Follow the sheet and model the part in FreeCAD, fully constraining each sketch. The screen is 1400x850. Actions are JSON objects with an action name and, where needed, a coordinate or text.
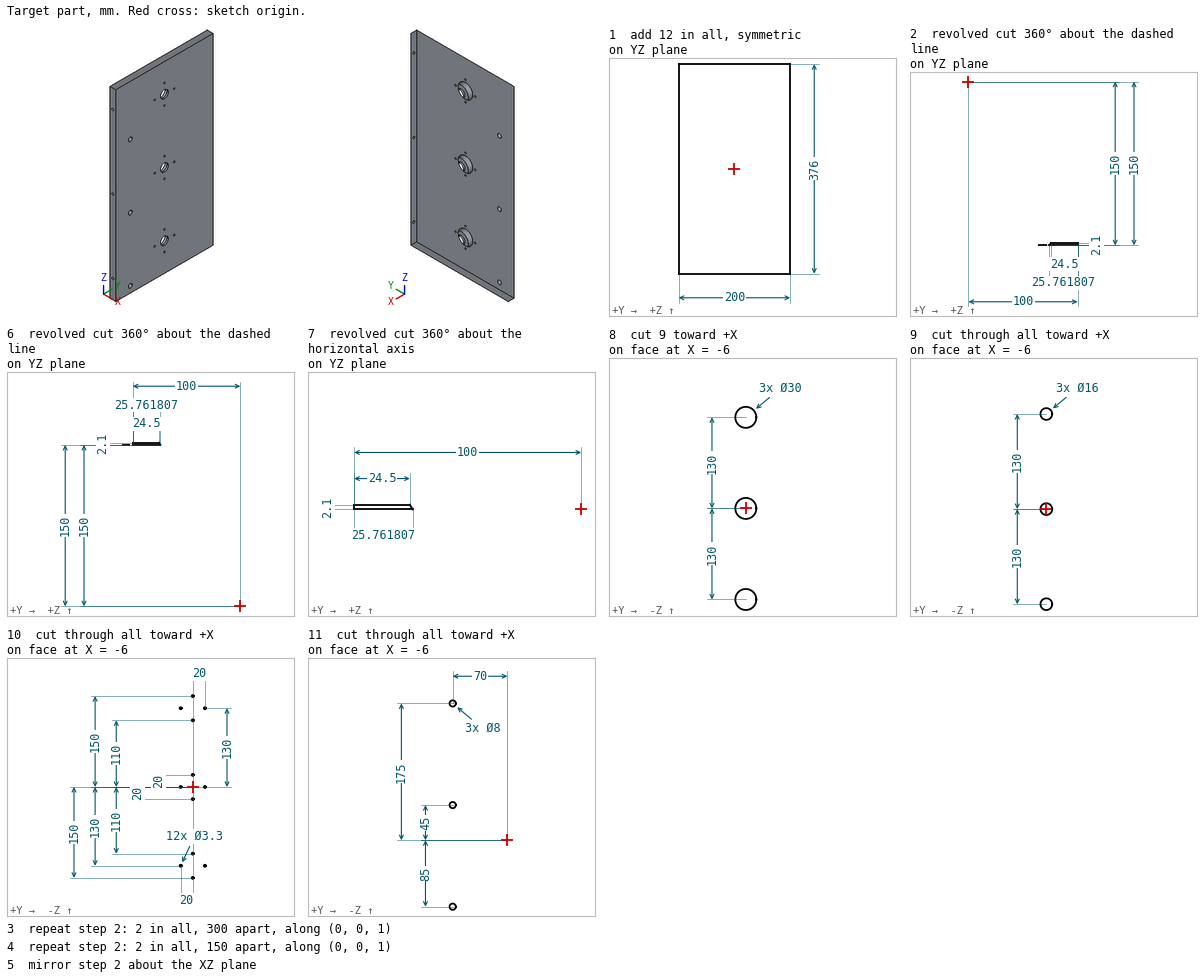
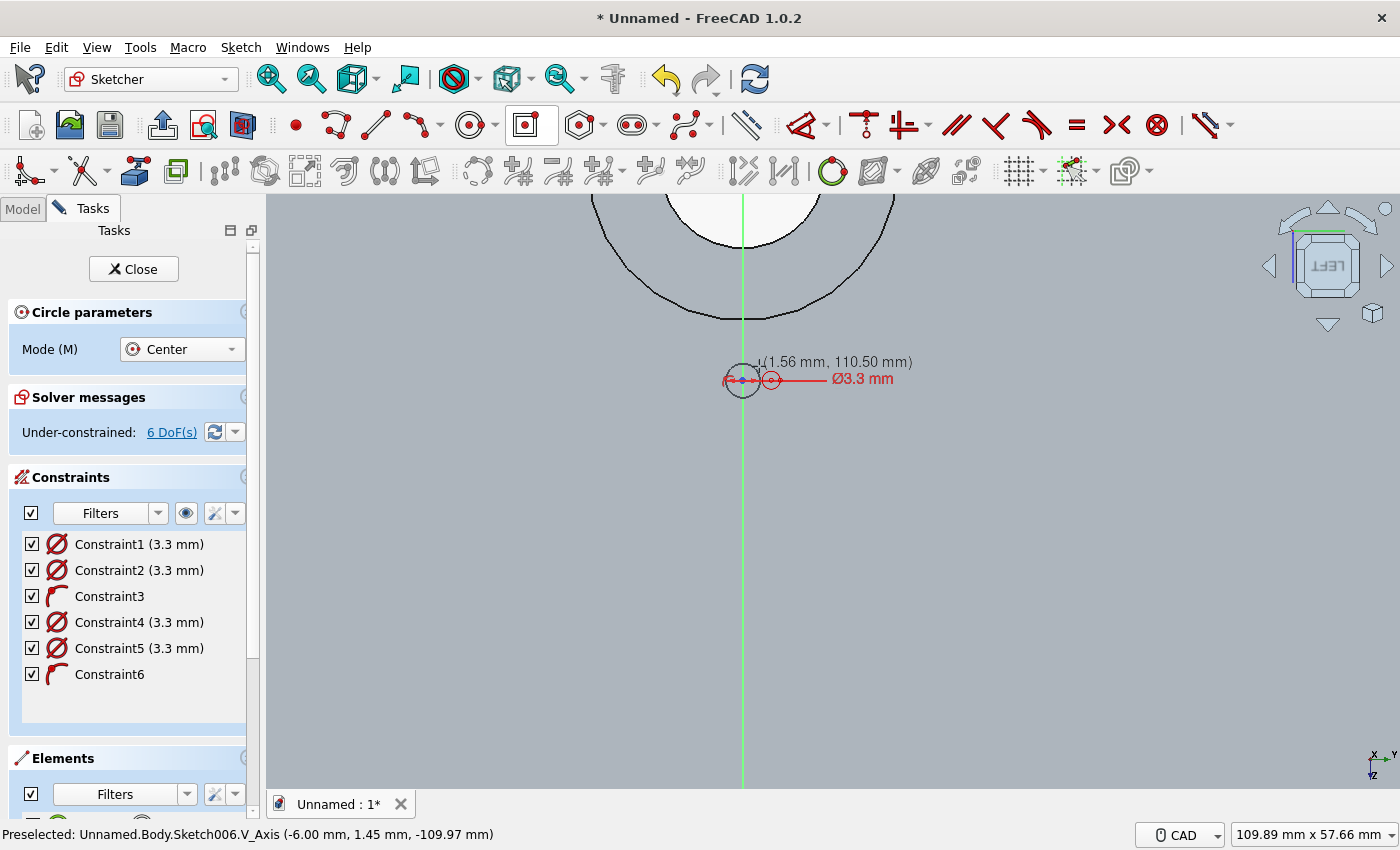
{"action": "scroll", "coordinate": [767, 365], "scroll_direction": "down", "scroll_amount": 11}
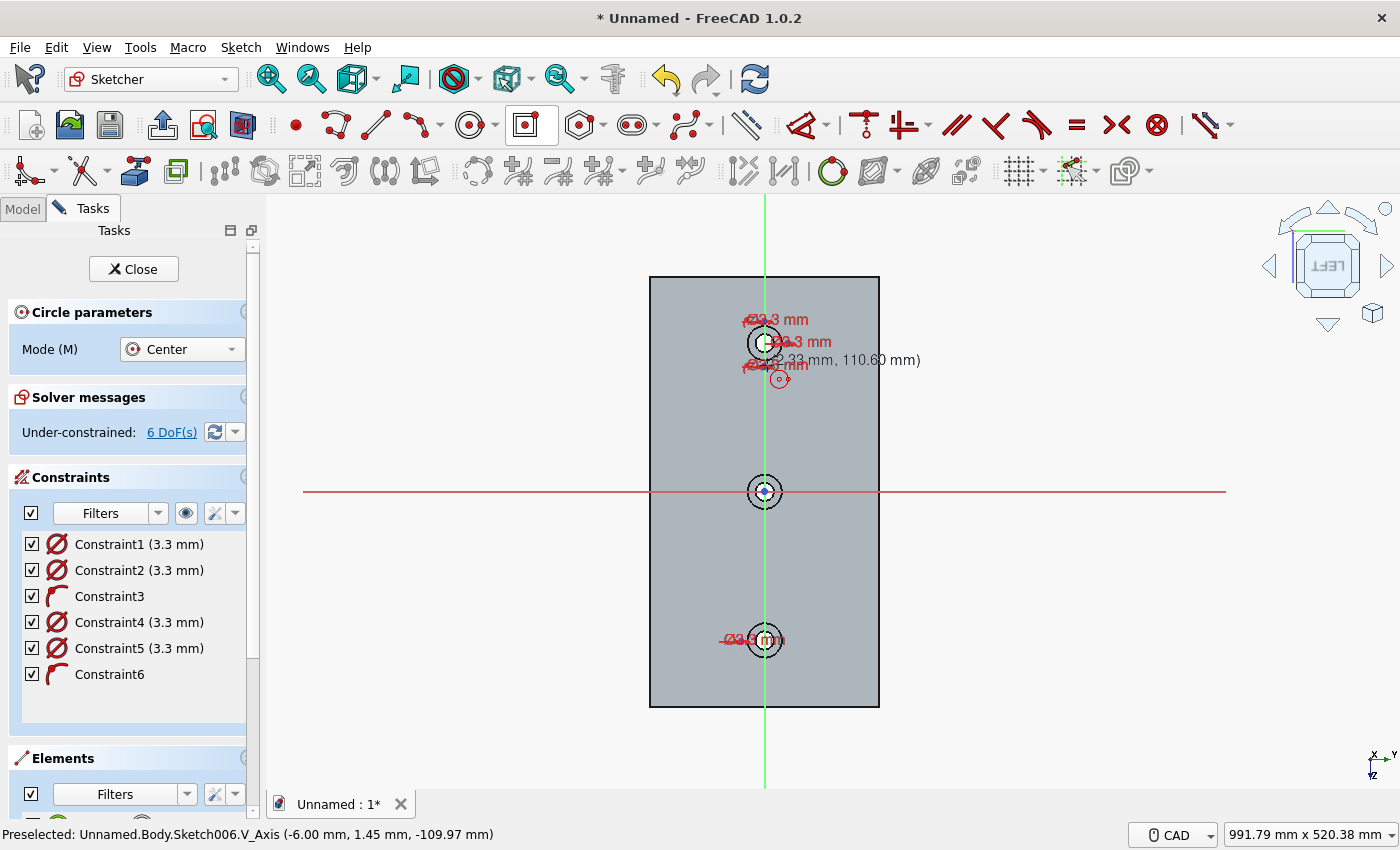
{"action": "scroll", "coordinate": [742, 343], "scroll_direction": "up", "scroll_amount": 13}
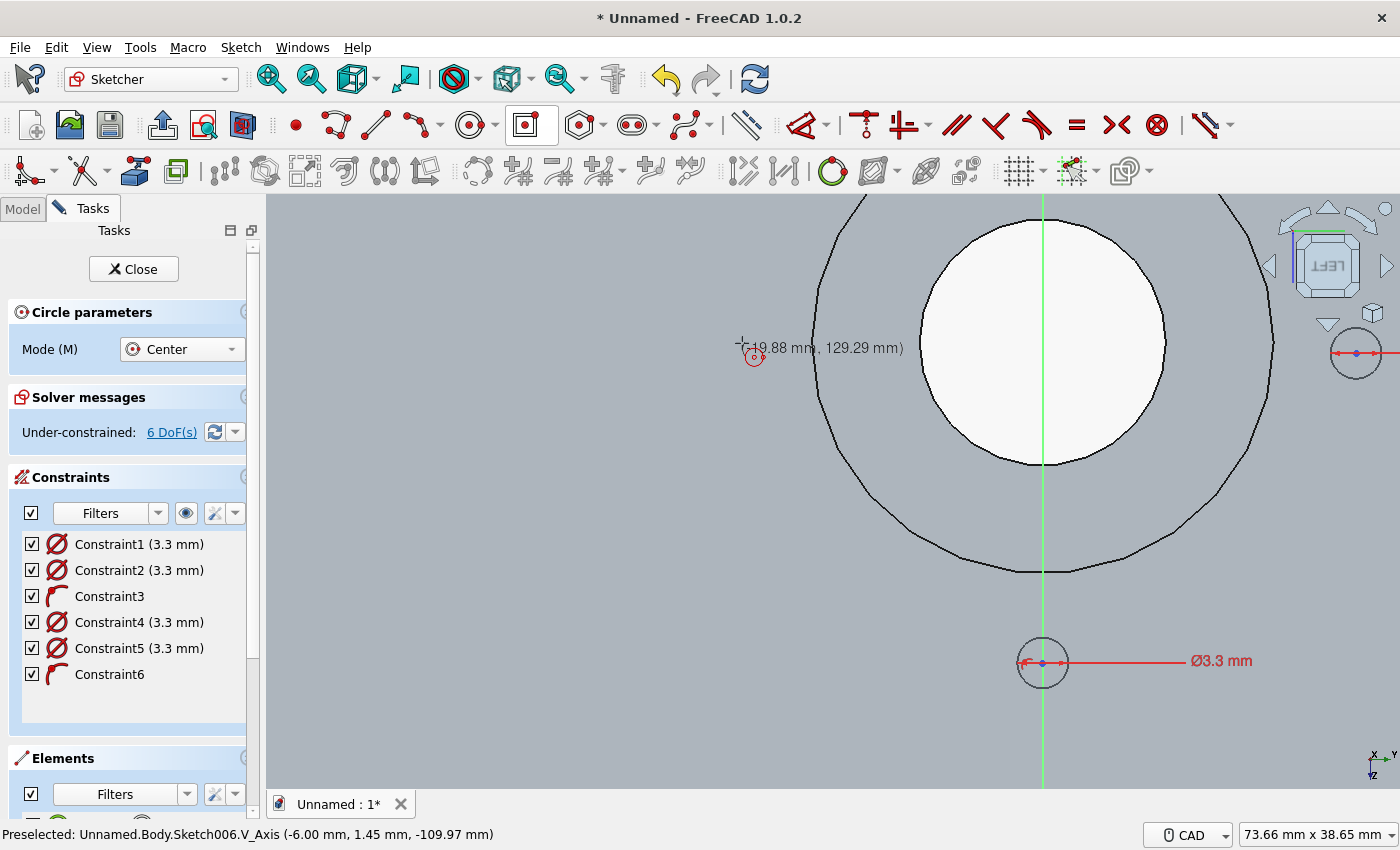
{"action": "scroll", "coordinate": [742, 343], "scroll_direction": "down", "scroll_amount": 13}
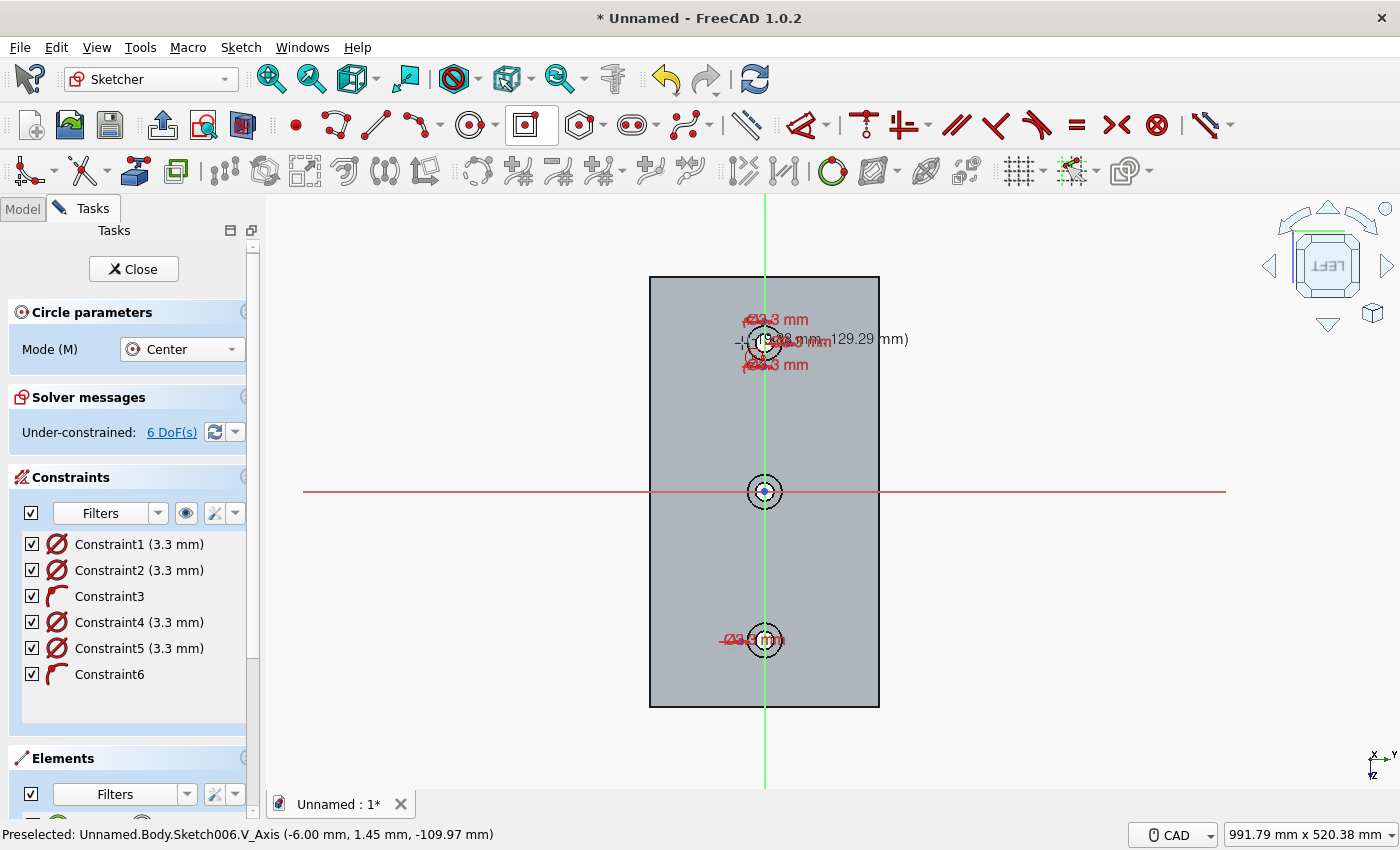
{"action": "left_click", "coordinate": [742, 343]}
{"action": "mouse_move", "coordinate": [743, 342]}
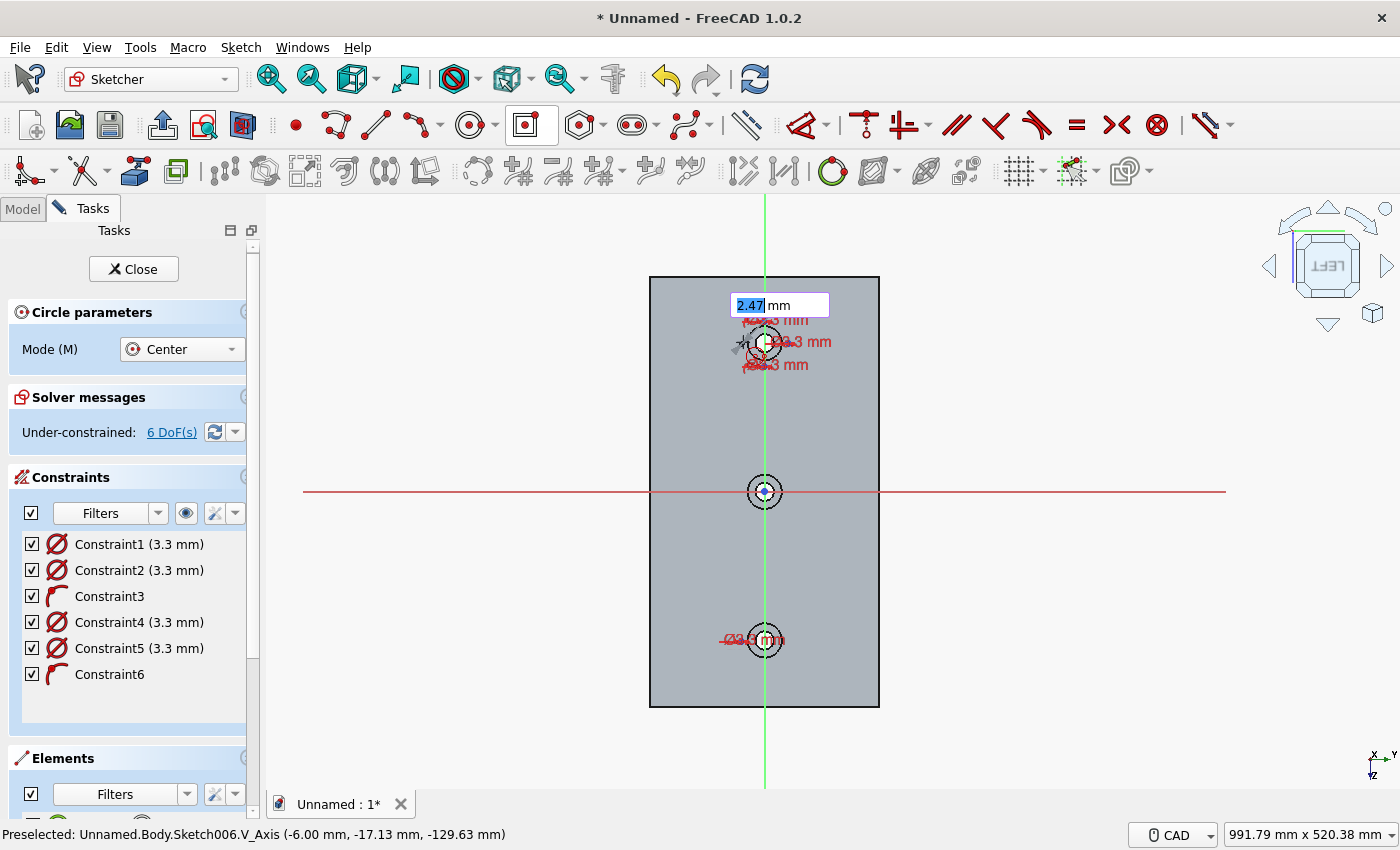
{"action": "type", "text": "3.3"}
{"action": "key", "text": "Return"}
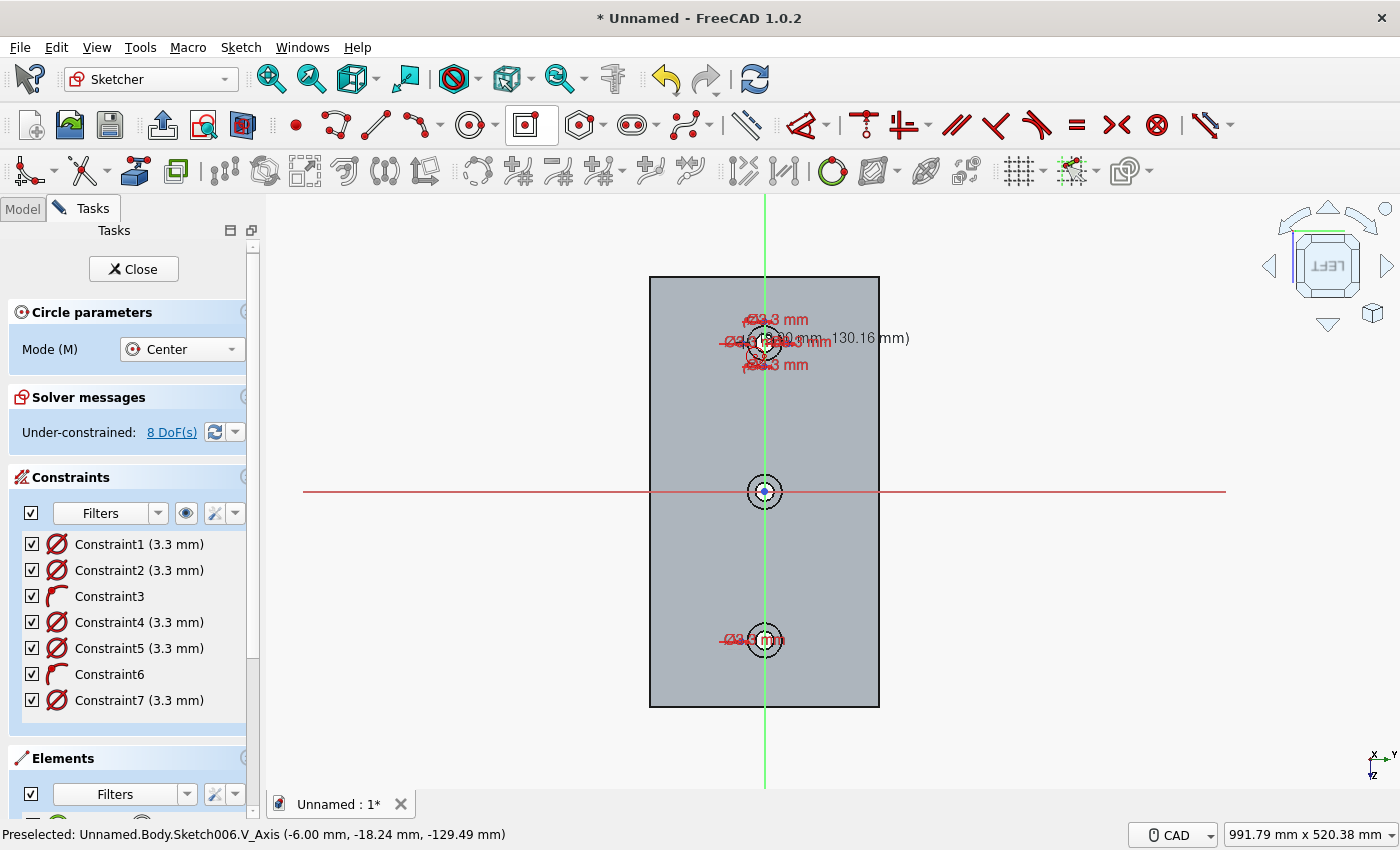
{"action": "scroll", "coordinate": [765, 469], "scroll_direction": "up", "scroll_amount": 13}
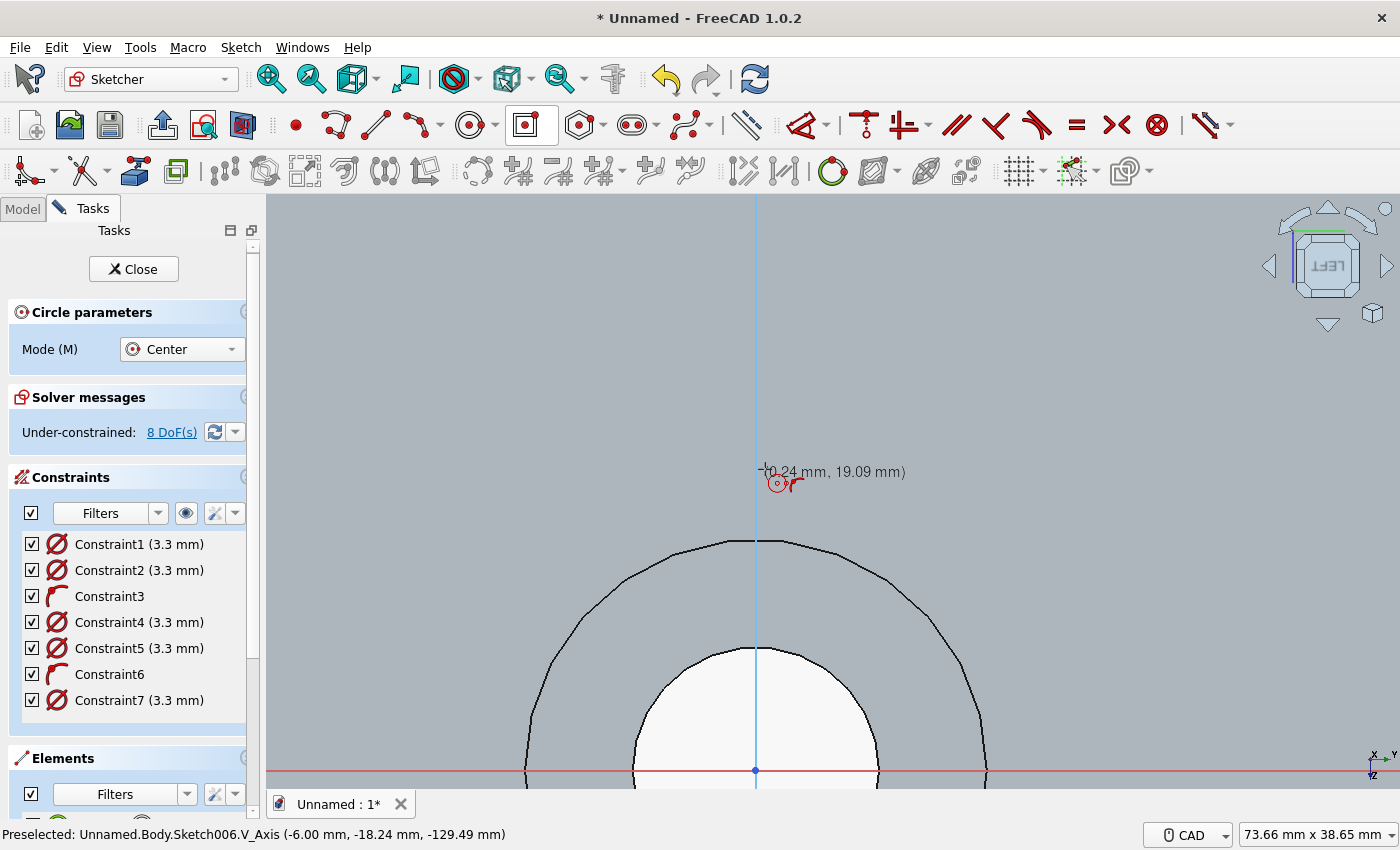
{"action": "scroll", "coordinate": [765, 469], "scroll_direction": "down", "scroll_amount": 13}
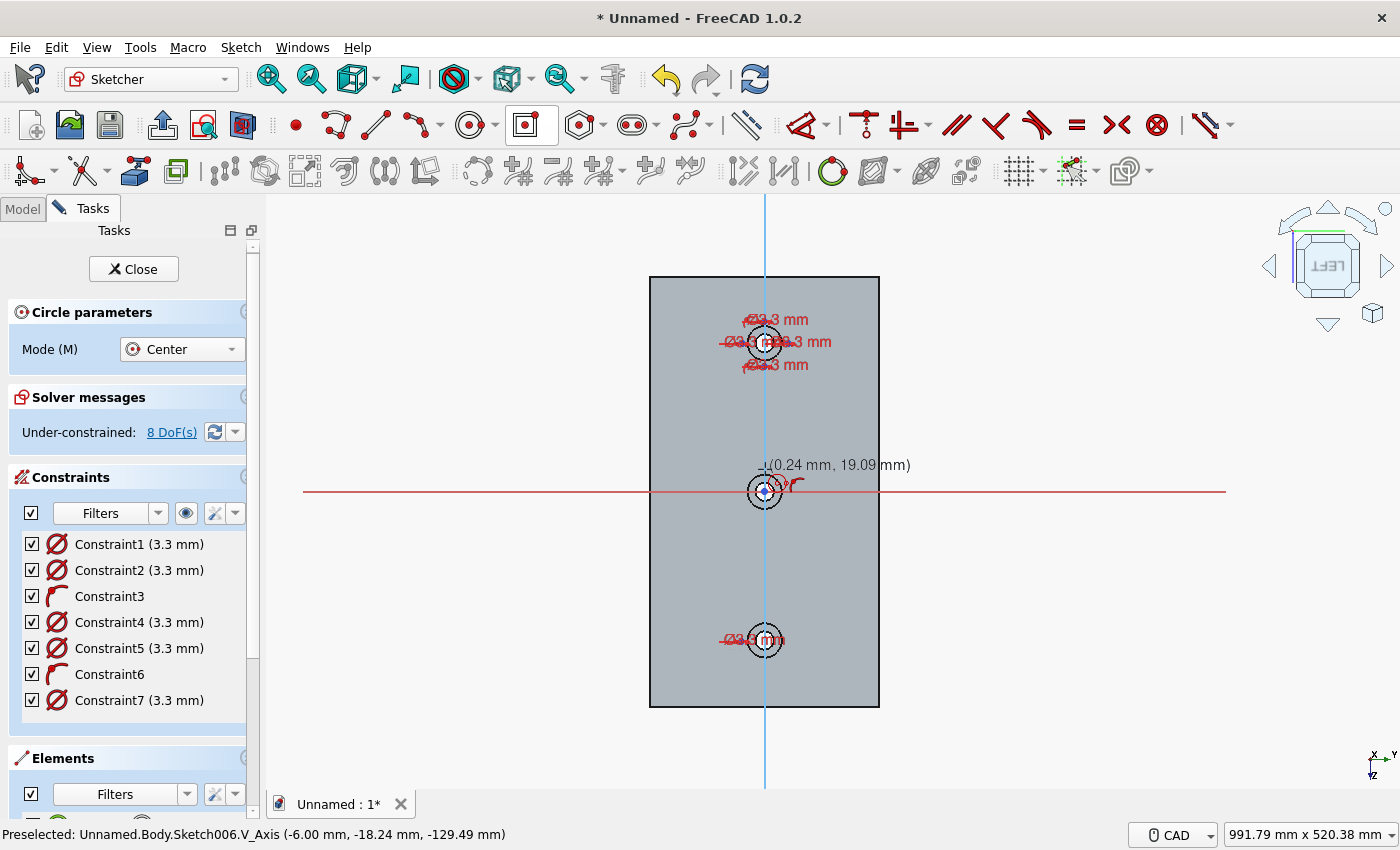
{"action": "left_click", "coordinate": [765, 469]}